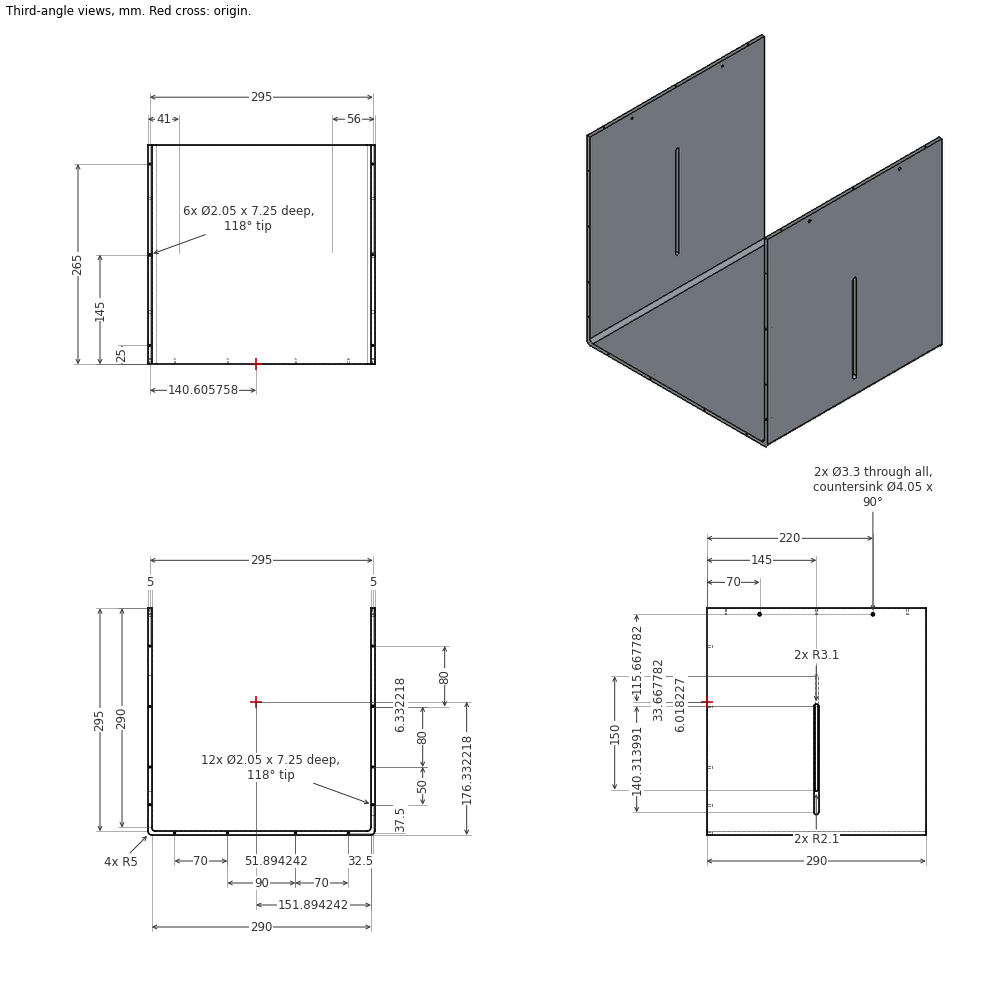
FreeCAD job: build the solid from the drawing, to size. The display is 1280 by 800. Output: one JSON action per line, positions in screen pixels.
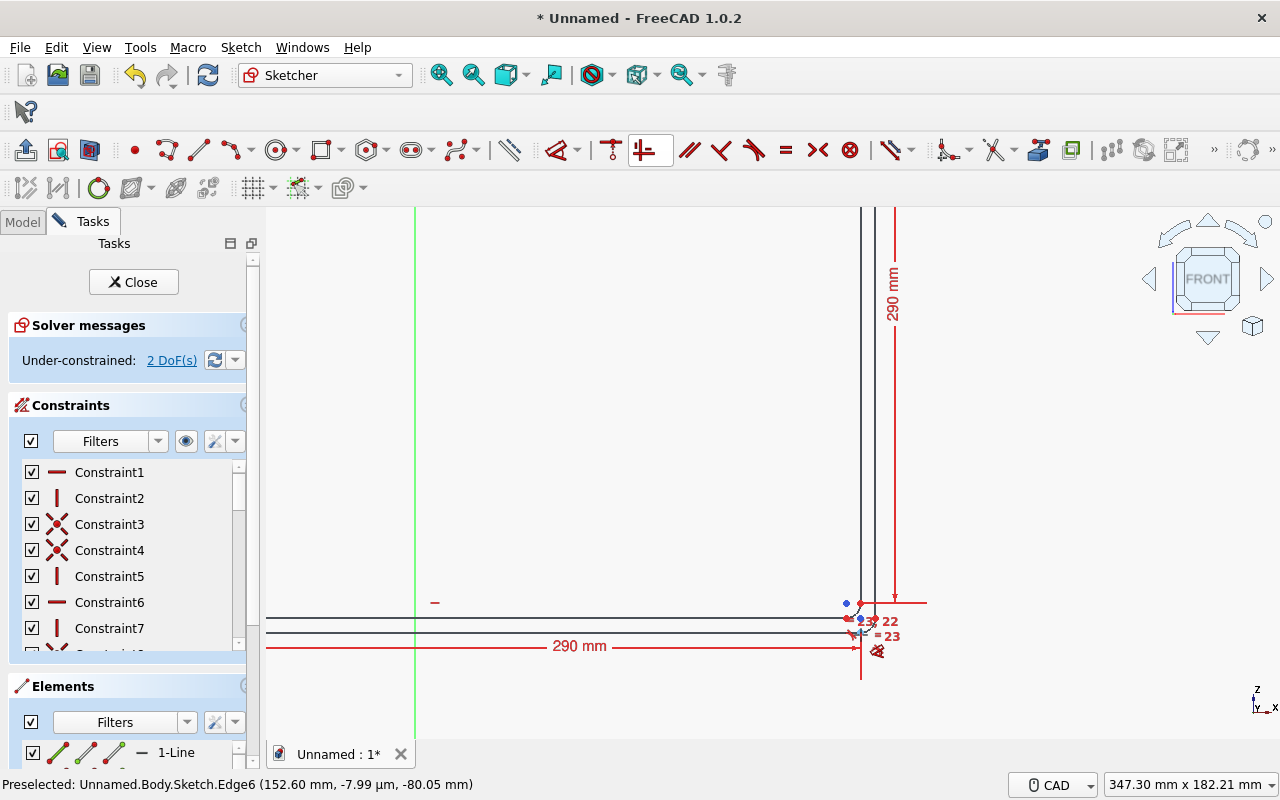
{"action": "left_click", "coordinate": [861, 633]}
{"action": "left_click", "coordinate": [638, 667]}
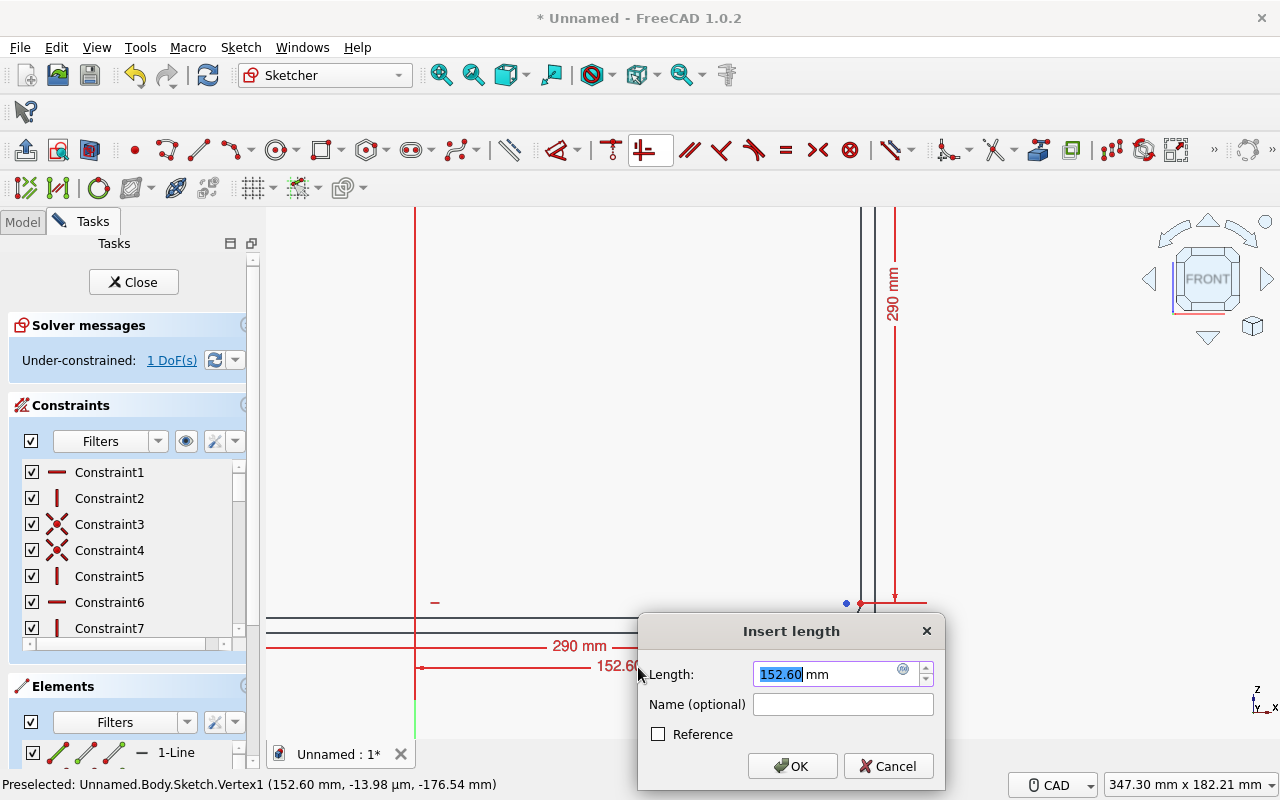
{"action": "type", "text": "151.894242"}
{"action": "key", "text": "Return"}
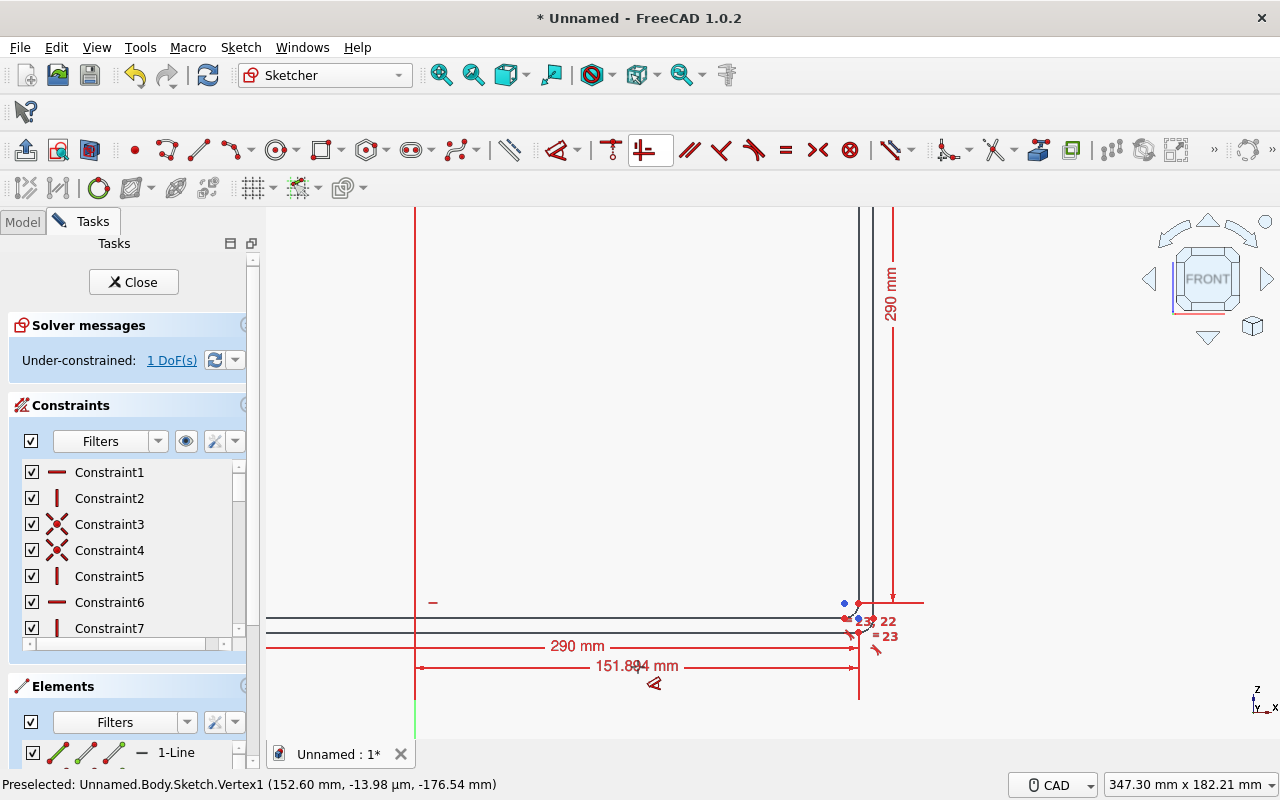
{"action": "left_click", "coordinate": [859, 633]}
{"action": "left_click", "coordinate": [893, 434]}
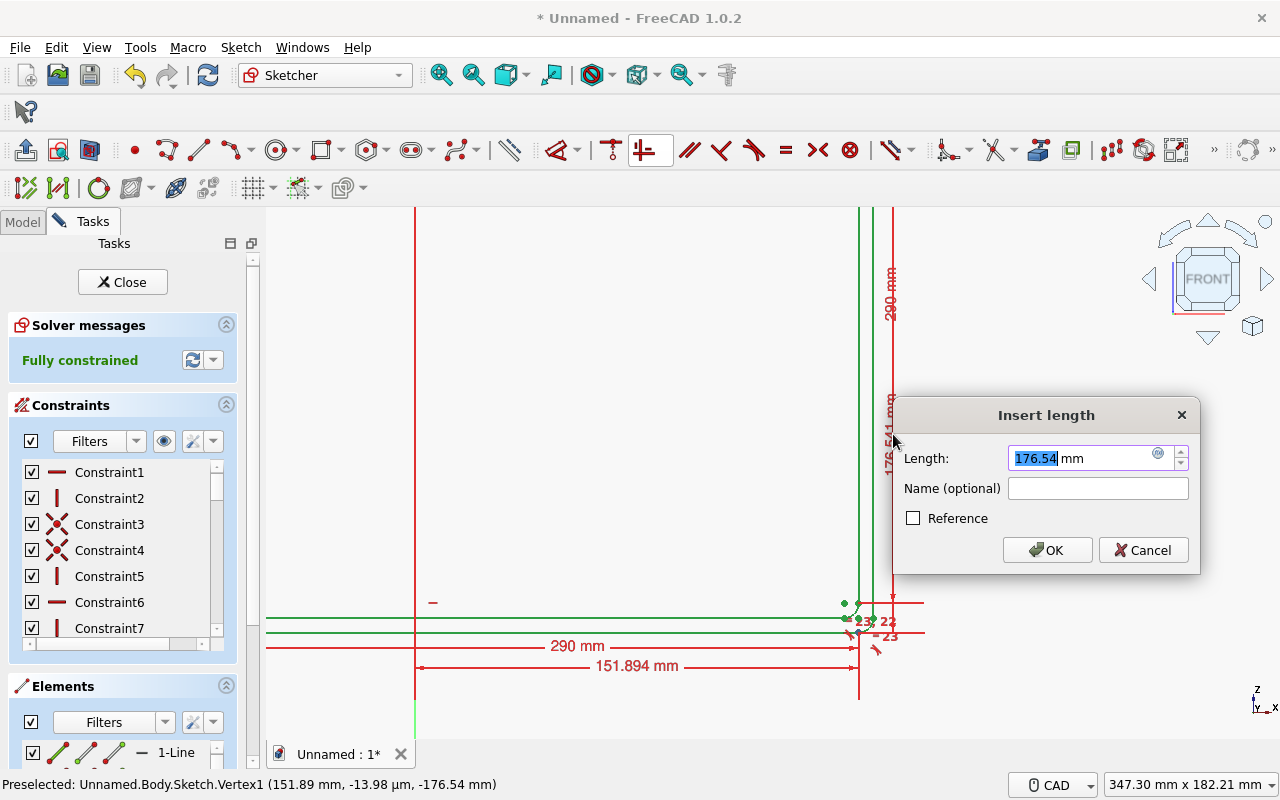
{"action": "type", "text": "176.332218"}
{"action": "key", "text": "Return"}
{"action": "key", "text": "Escape"}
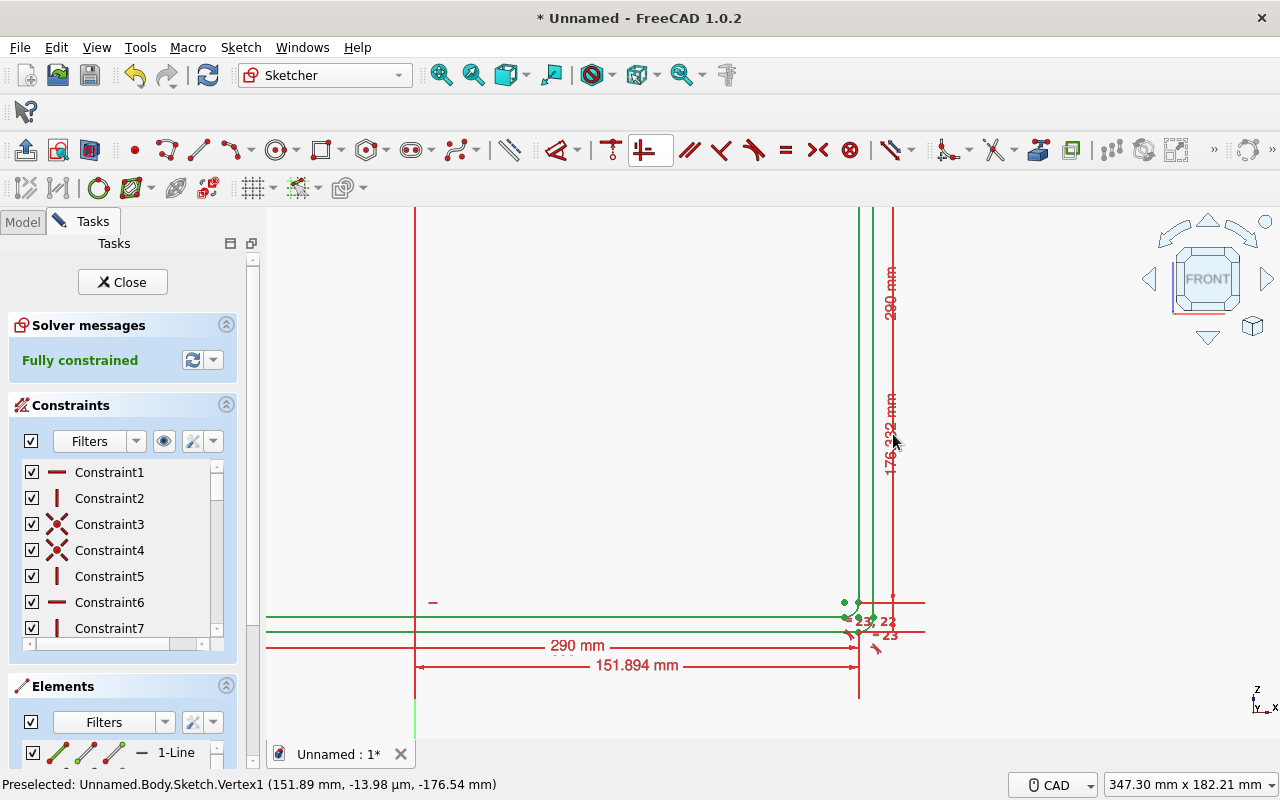
{"action": "left_click", "coordinate": [123, 282]}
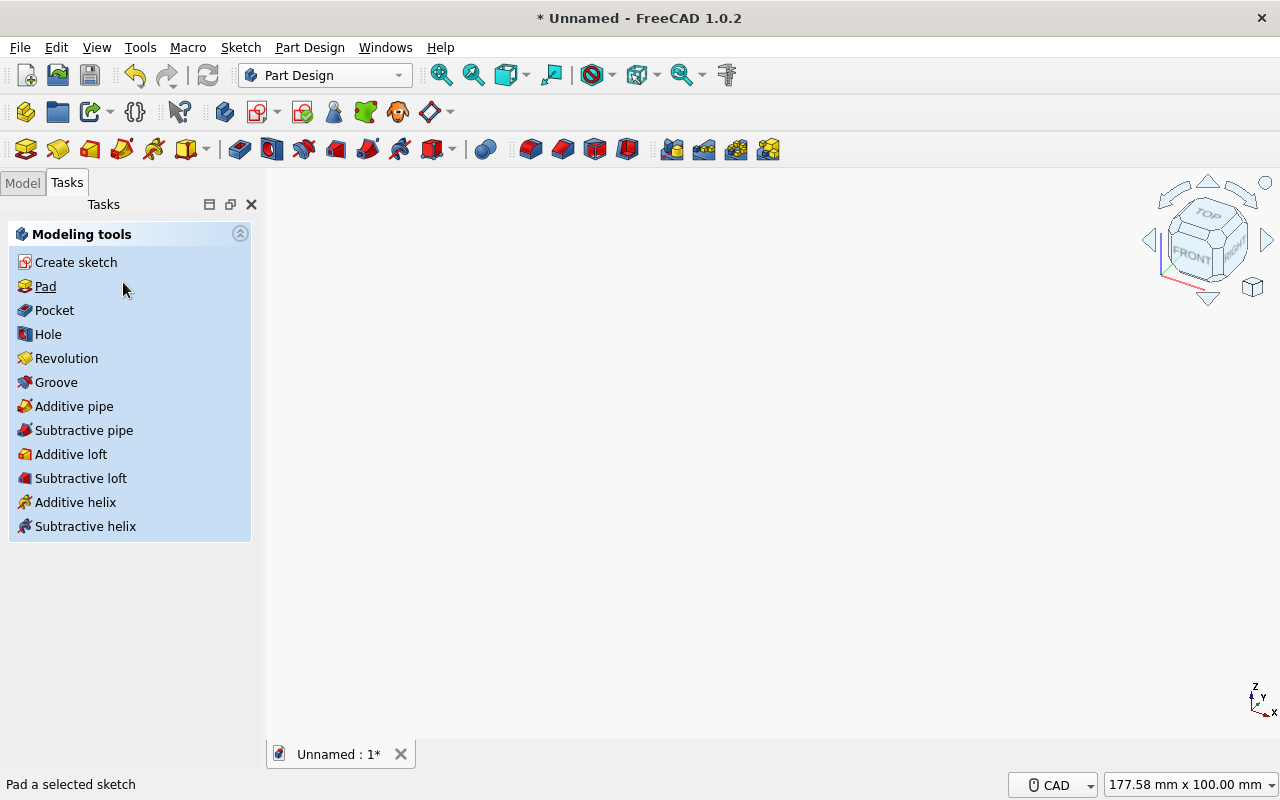
{"action": "left_click", "coordinate": [26, 150]}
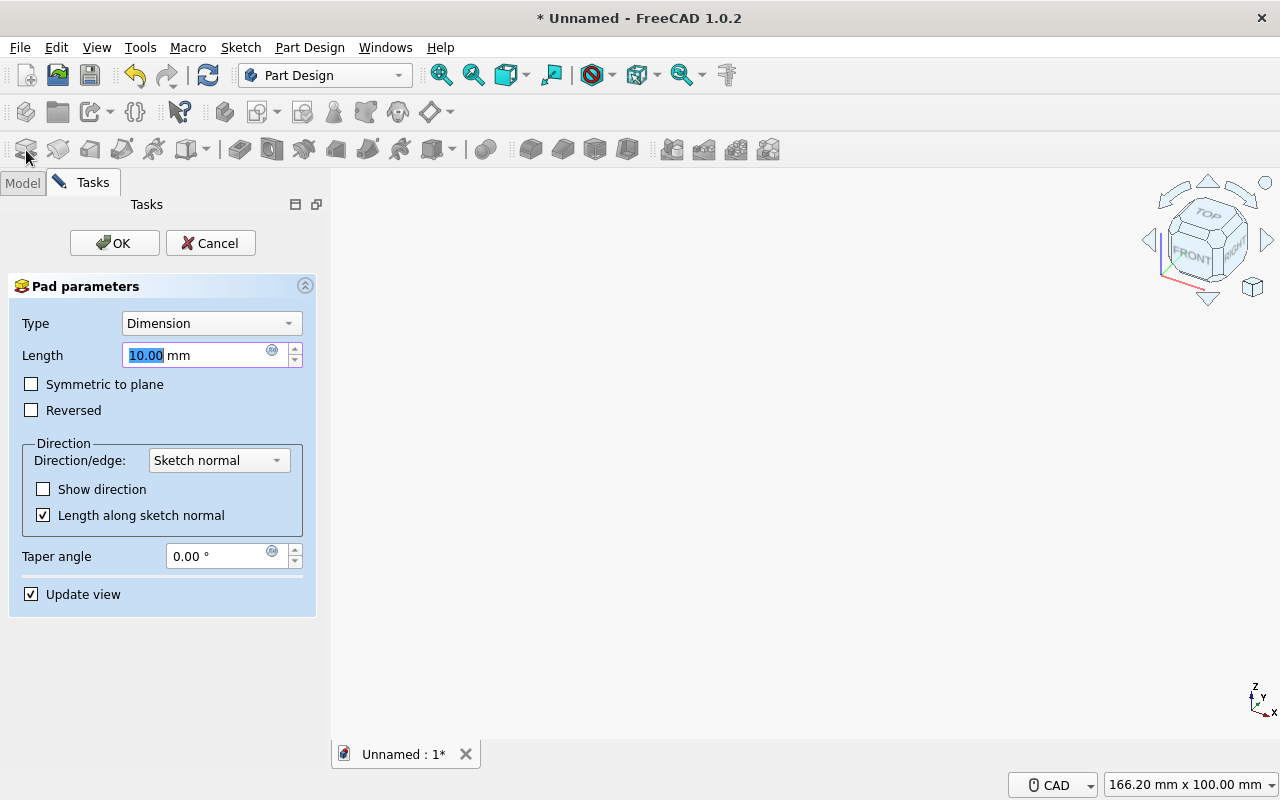
{"action": "type", "text": "290"}
{"action": "key", "text": "Tab"}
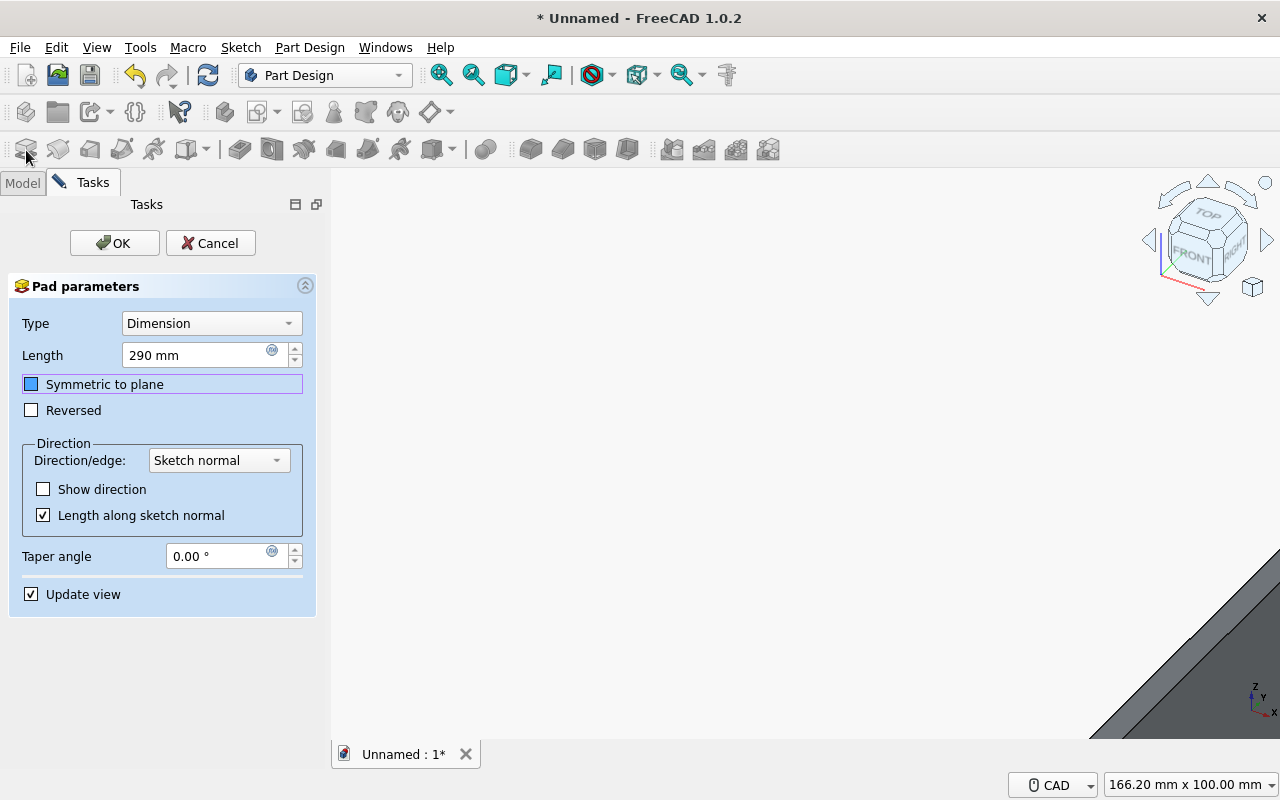
{"action": "left_click", "coordinate": [30, 410]}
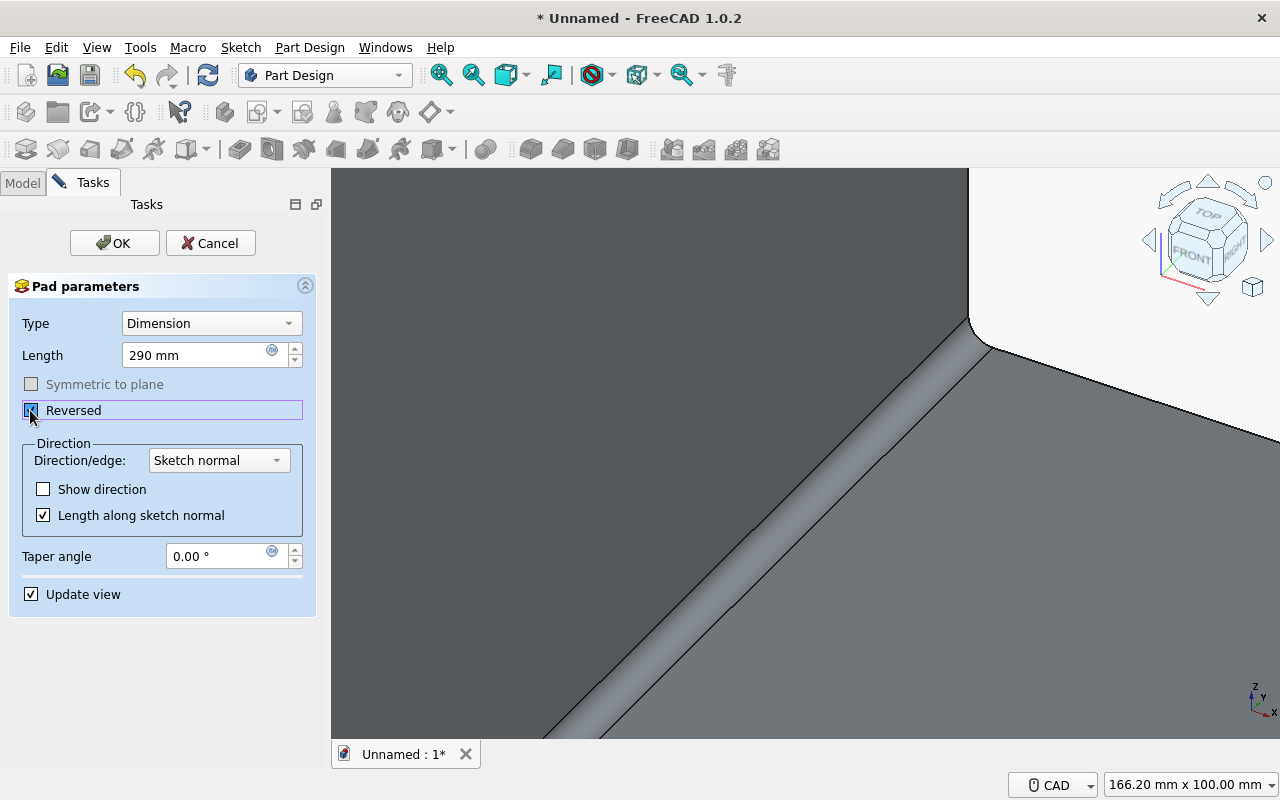
{"action": "left_click", "coordinate": [115, 243]}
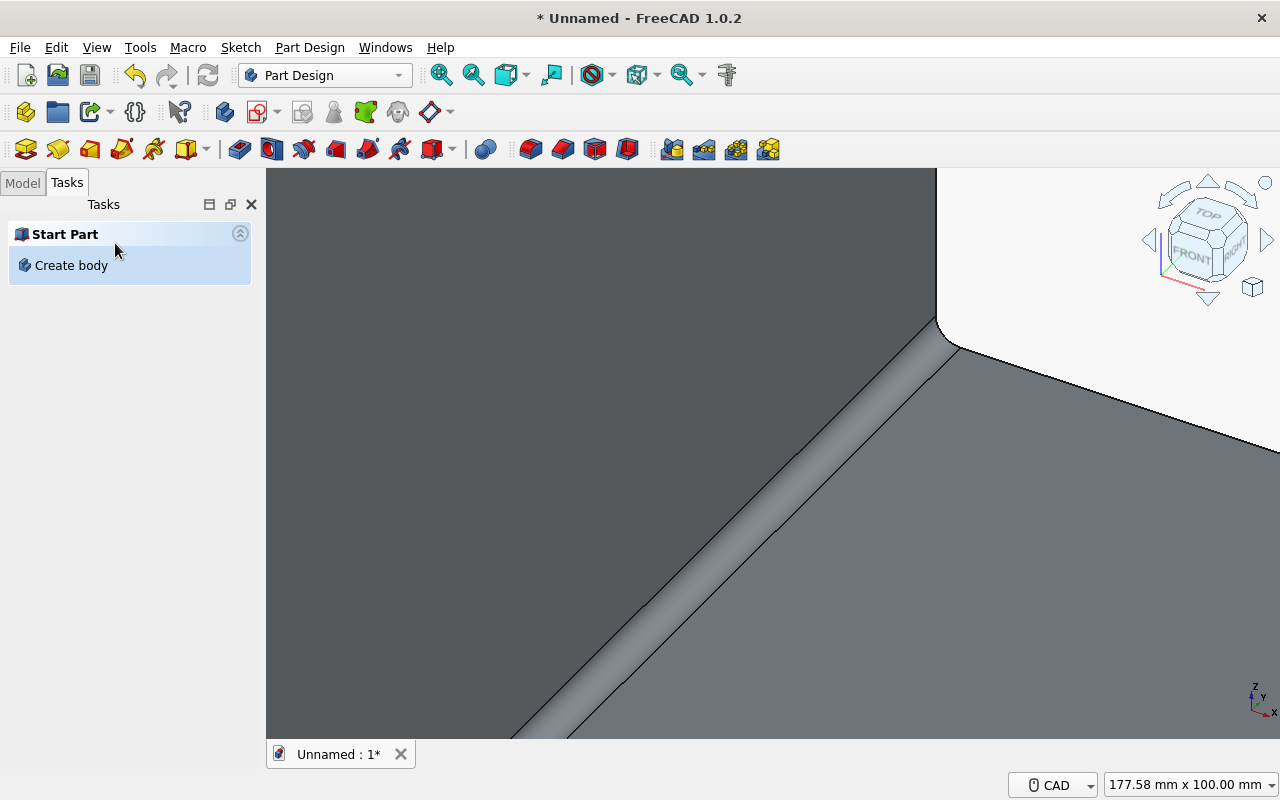
{"action": "left_click", "coordinate": [442, 76]}